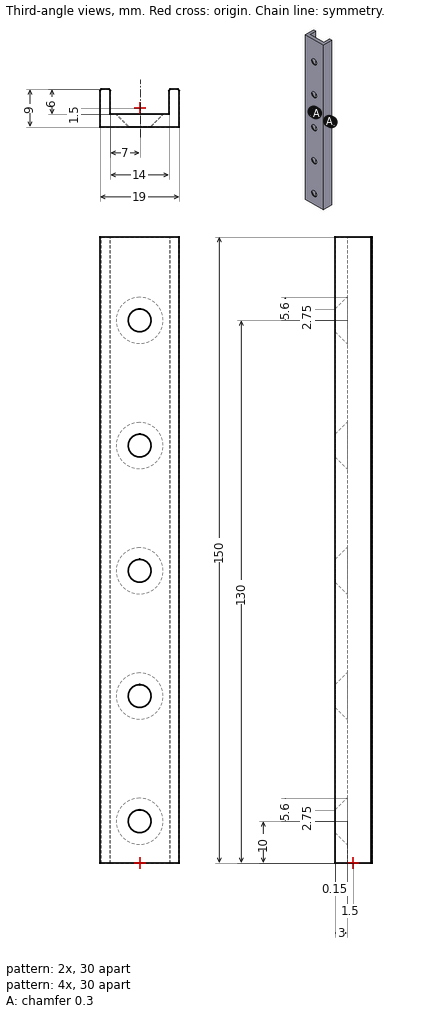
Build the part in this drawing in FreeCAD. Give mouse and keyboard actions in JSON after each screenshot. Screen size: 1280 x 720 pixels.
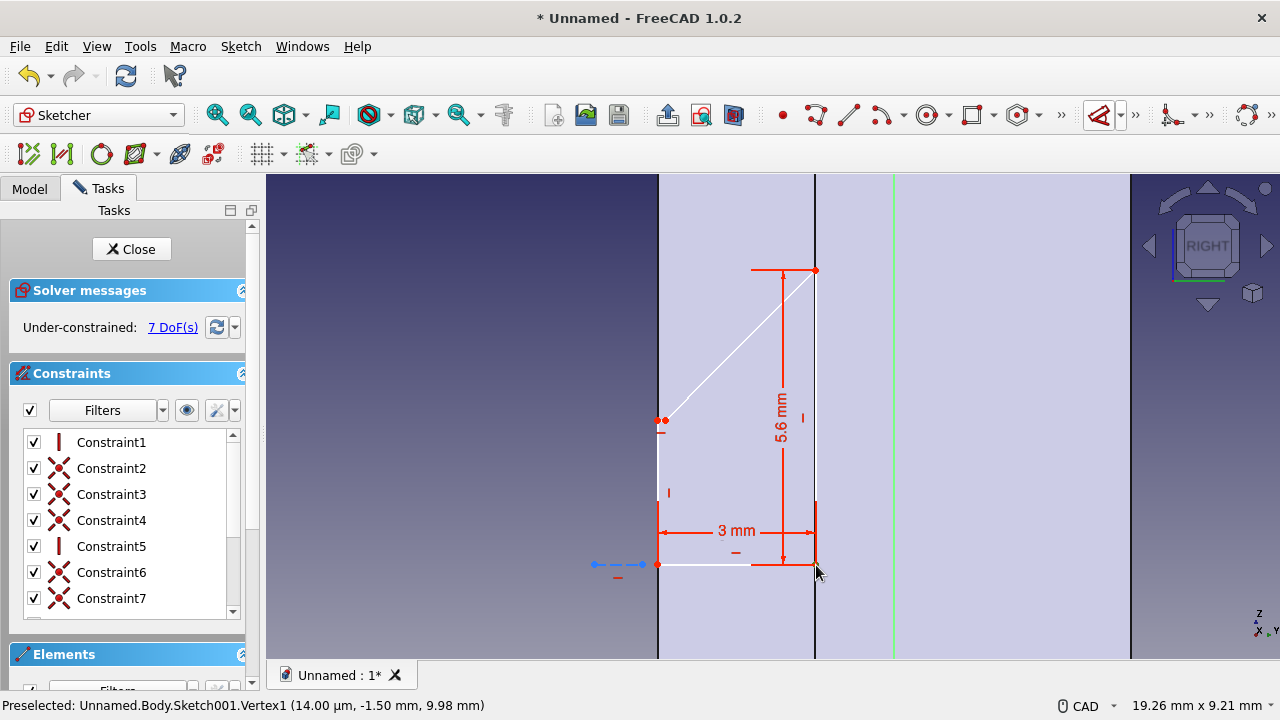
{"action": "key", "text": "i"}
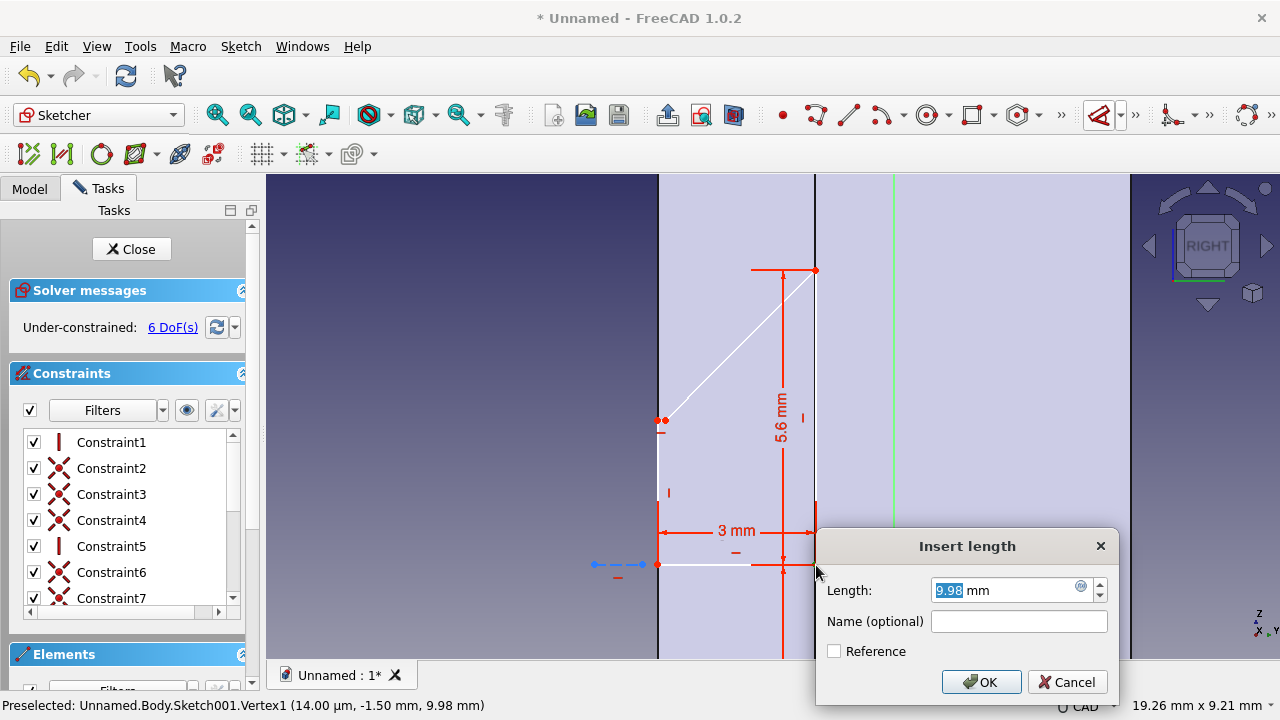
{"action": "type", "text": "10"}
{"action": "key", "text": "Return"}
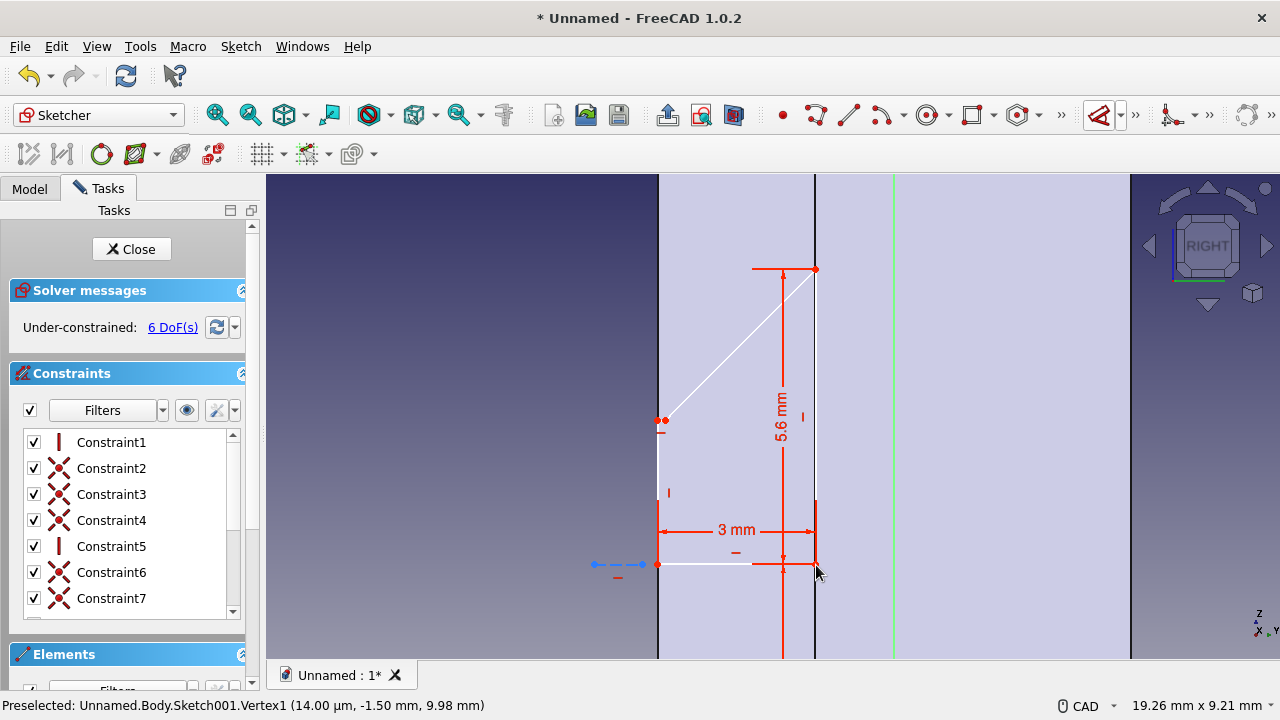
{"action": "left_click", "coordinate": [642, 565]}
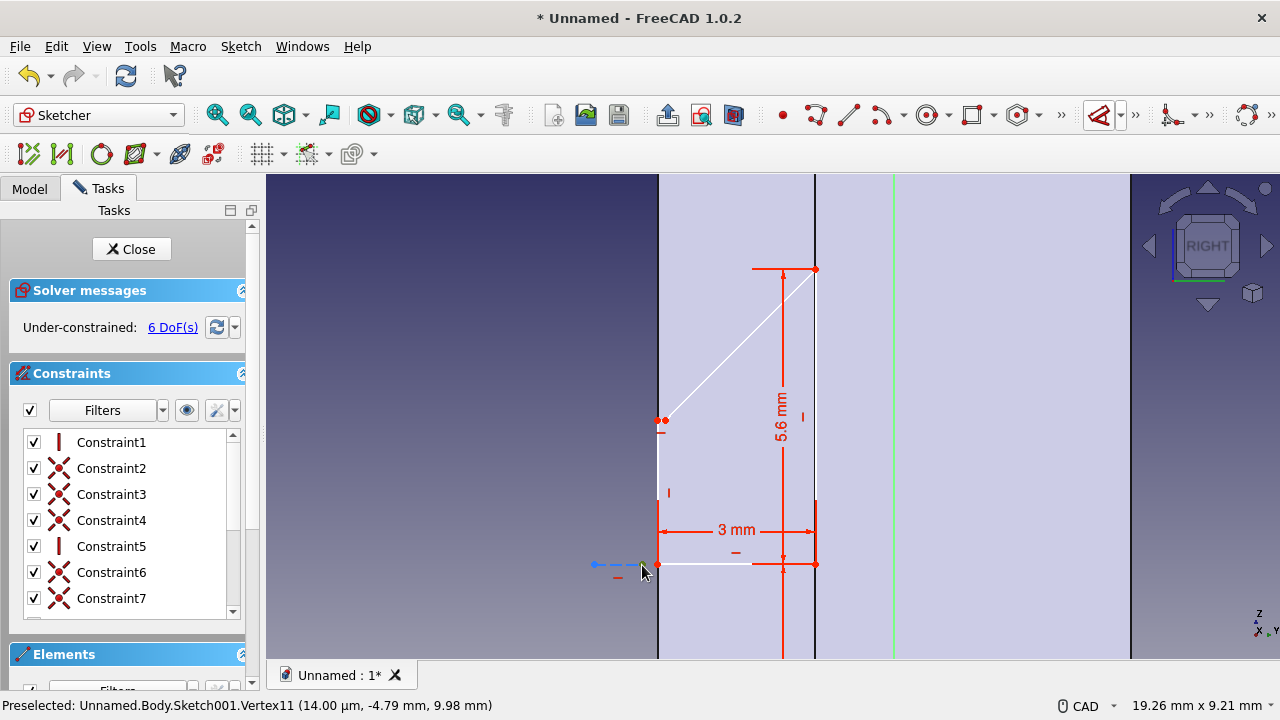
{"action": "key", "text": "i"}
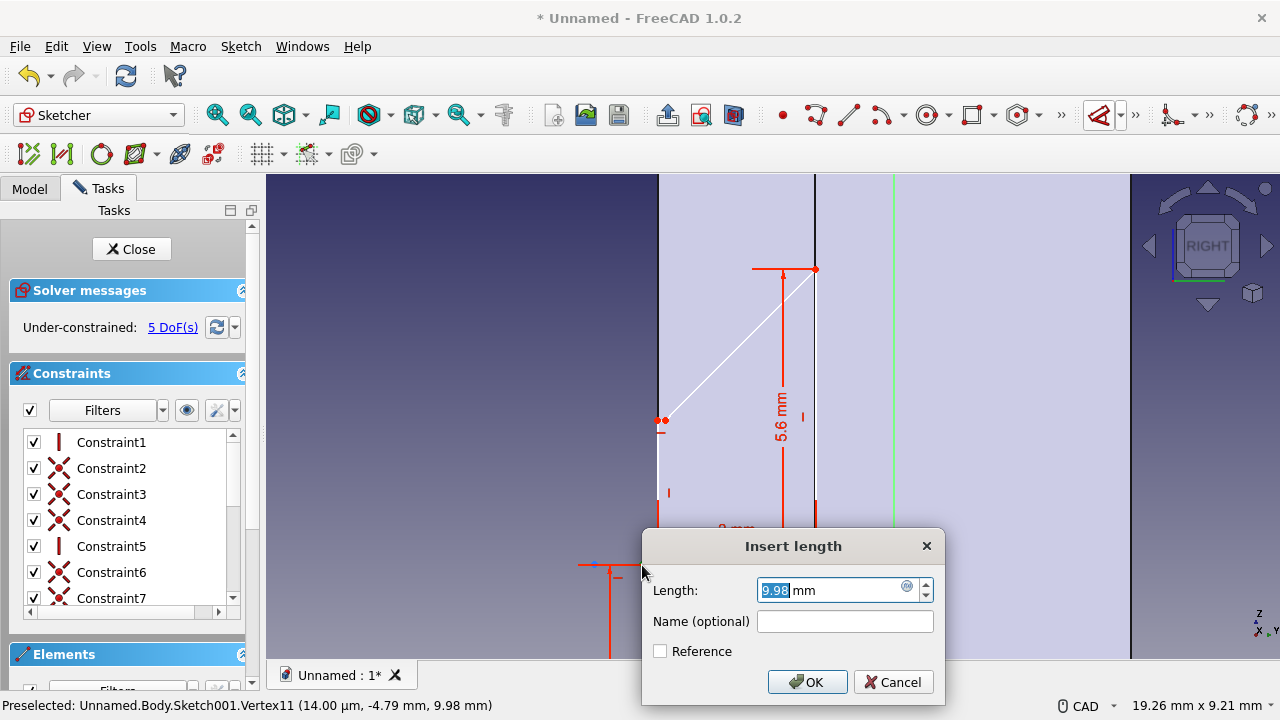
{"action": "type", "text": "10"}
{"action": "key", "text": "Return"}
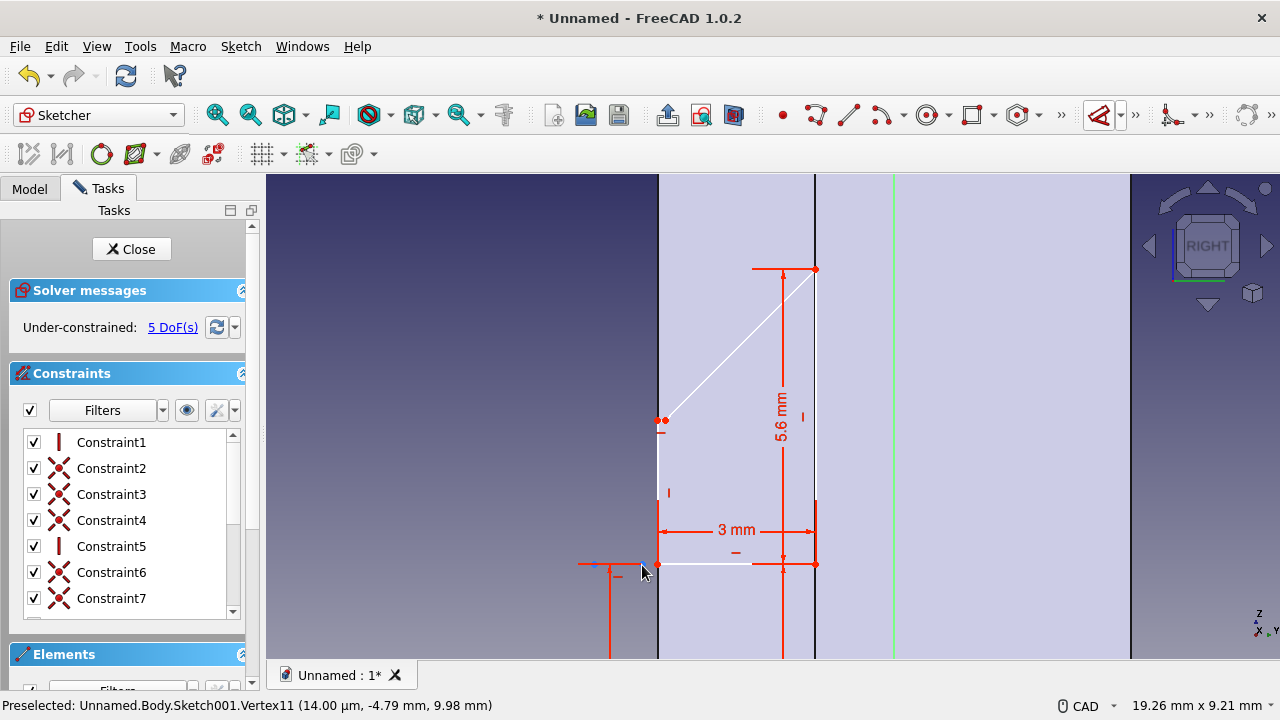
{"action": "scroll", "coordinate": [662, 421], "scroll_direction": "up", "scroll_amount": 9}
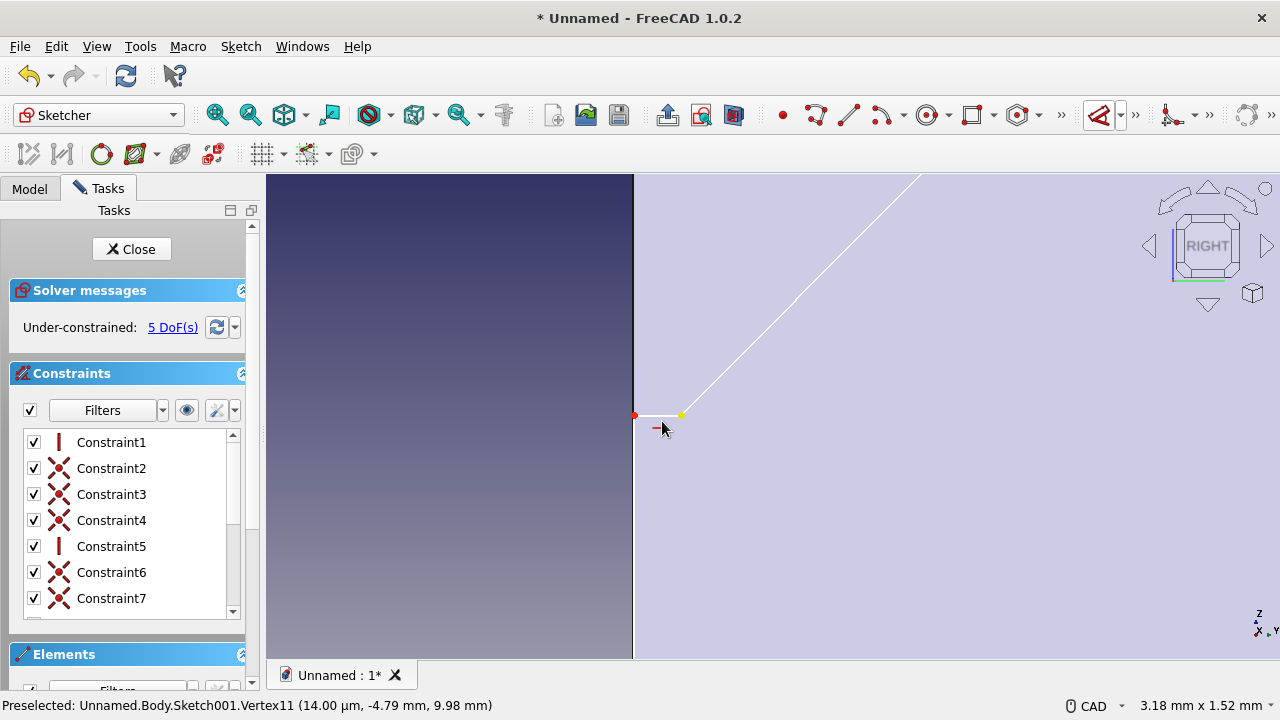
{"action": "left_click", "coordinate": [658, 416]}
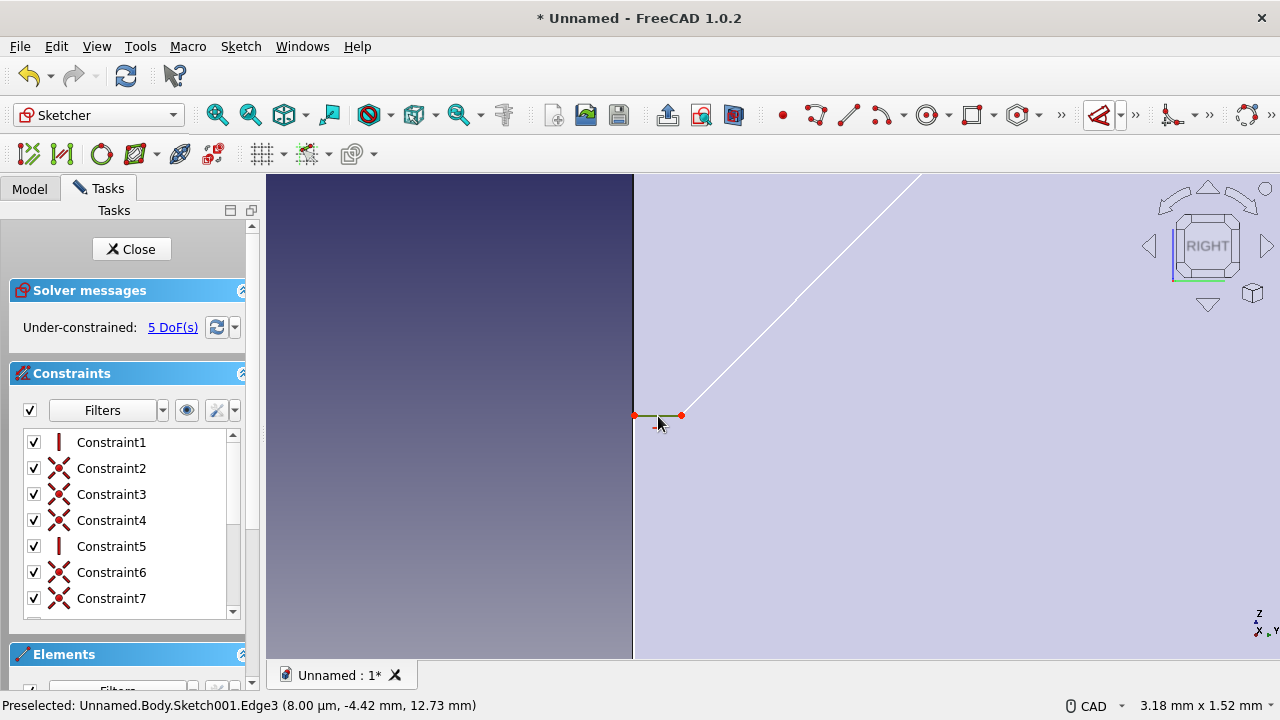
{"action": "key", "text": "l"}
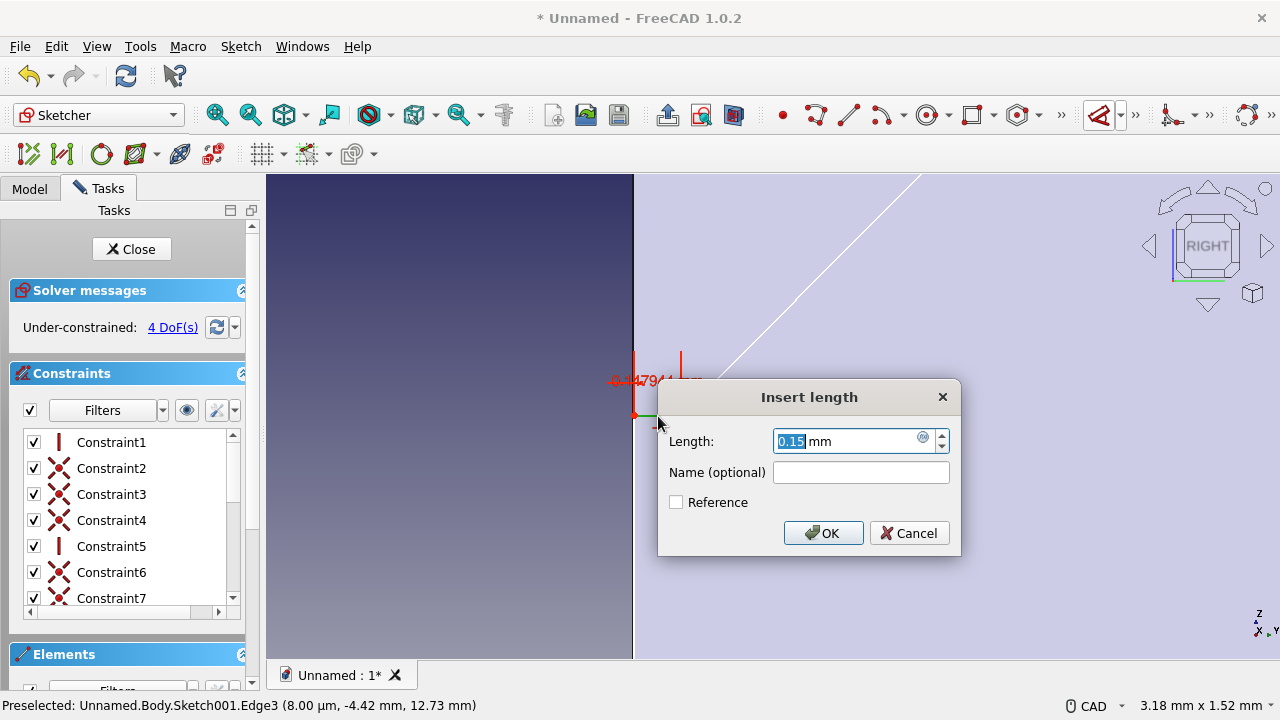
{"action": "type", "text": "0.15"}
{"action": "key", "text": "Return"}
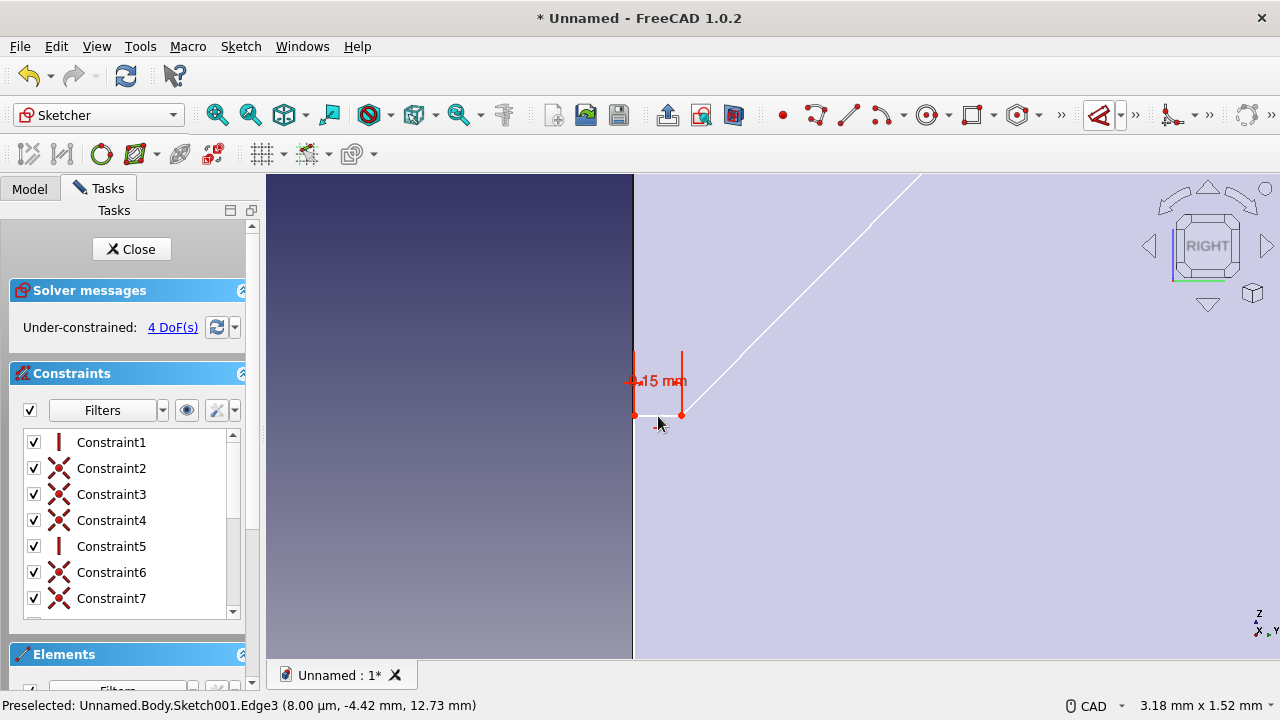
{"action": "scroll", "coordinate": [662, 421], "scroll_direction": "down", "scroll_amount": 9}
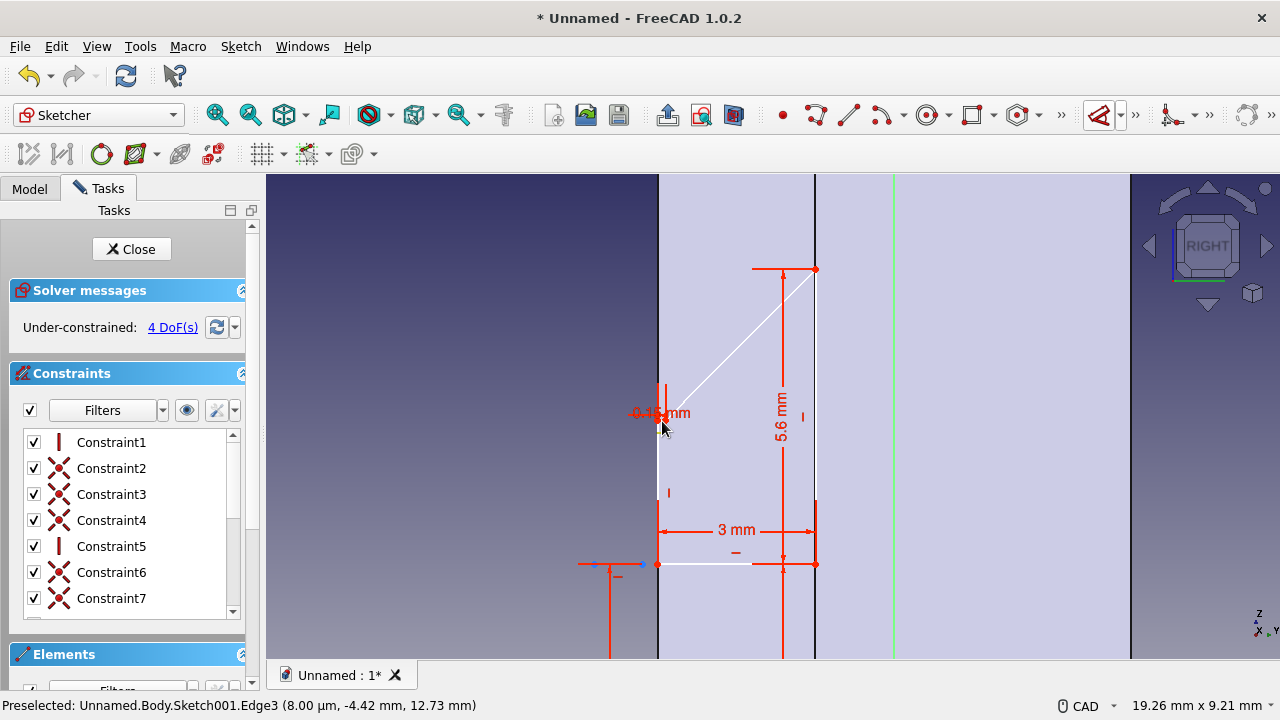
{"action": "left_click", "coordinate": [658, 449]}